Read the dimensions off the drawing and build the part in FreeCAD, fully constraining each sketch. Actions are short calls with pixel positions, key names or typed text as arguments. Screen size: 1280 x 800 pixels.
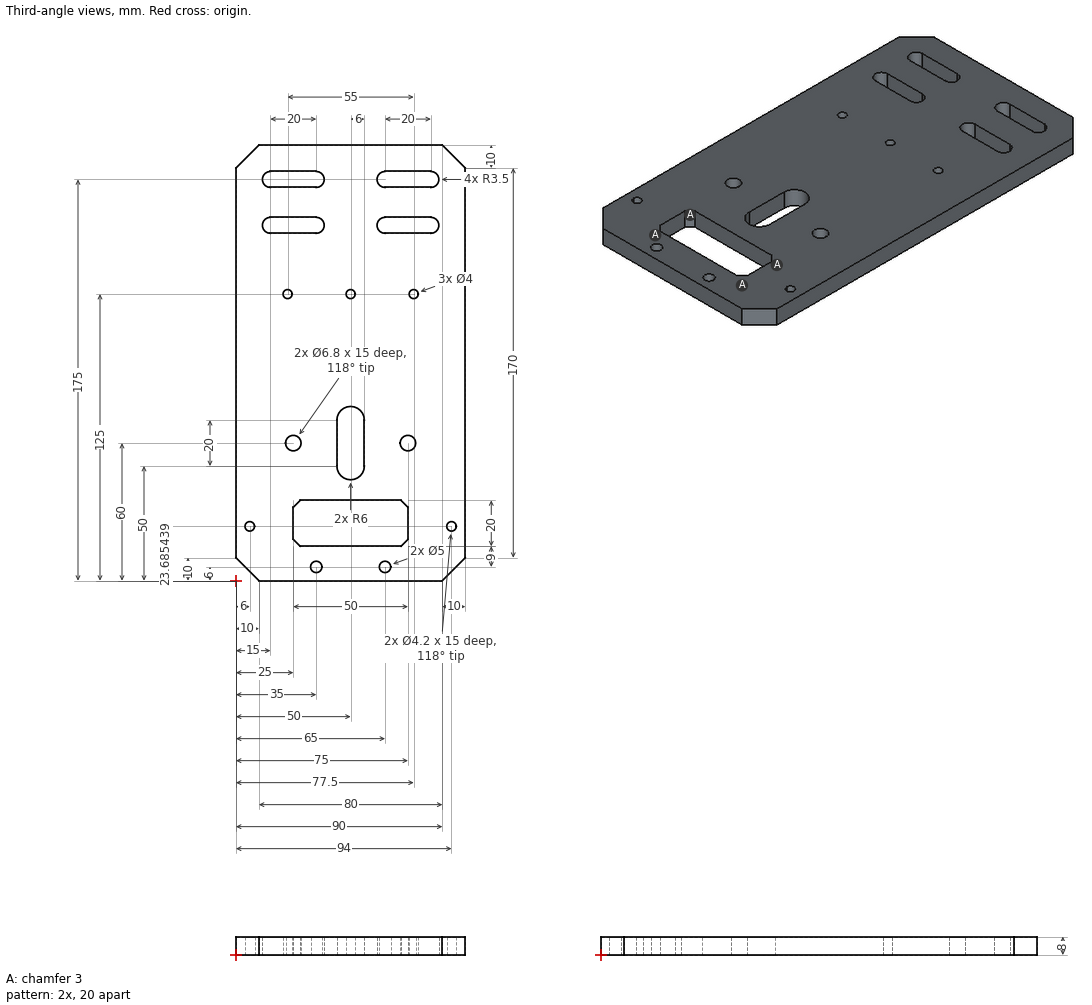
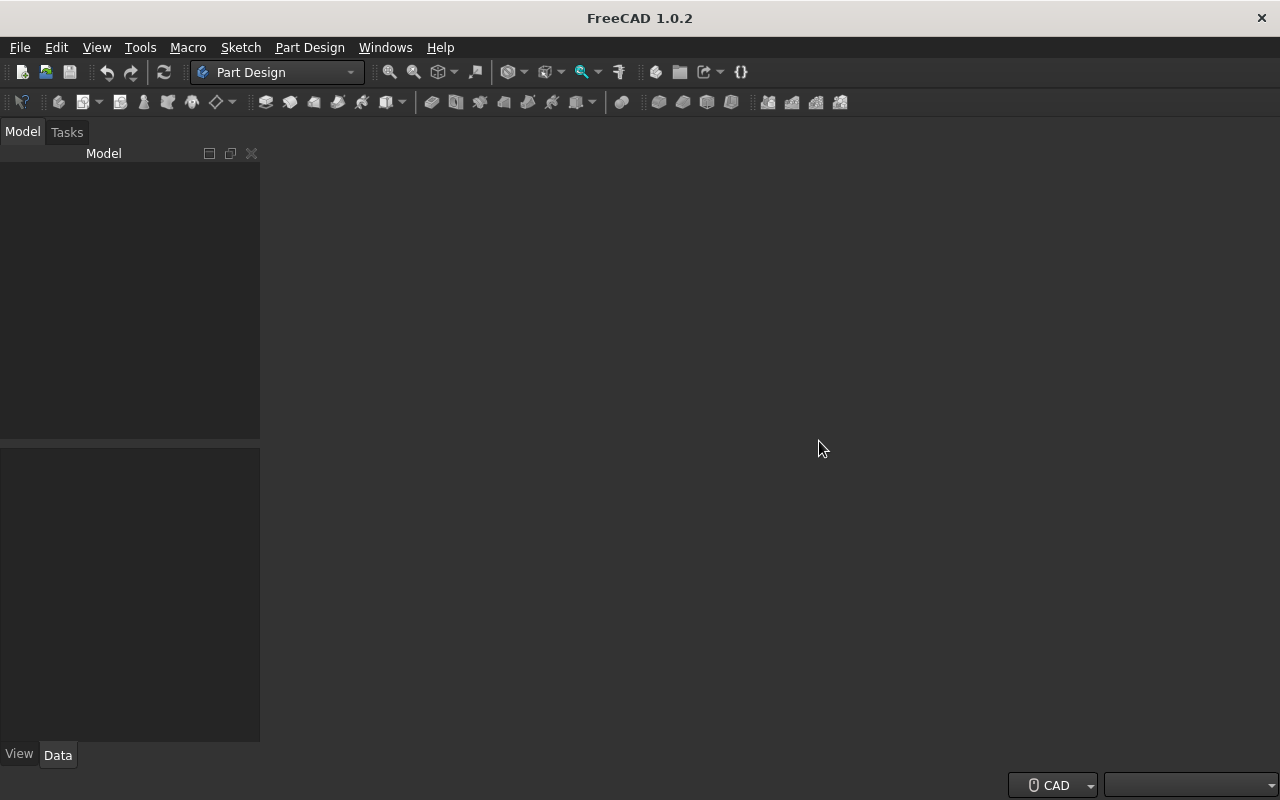
click(22, 72)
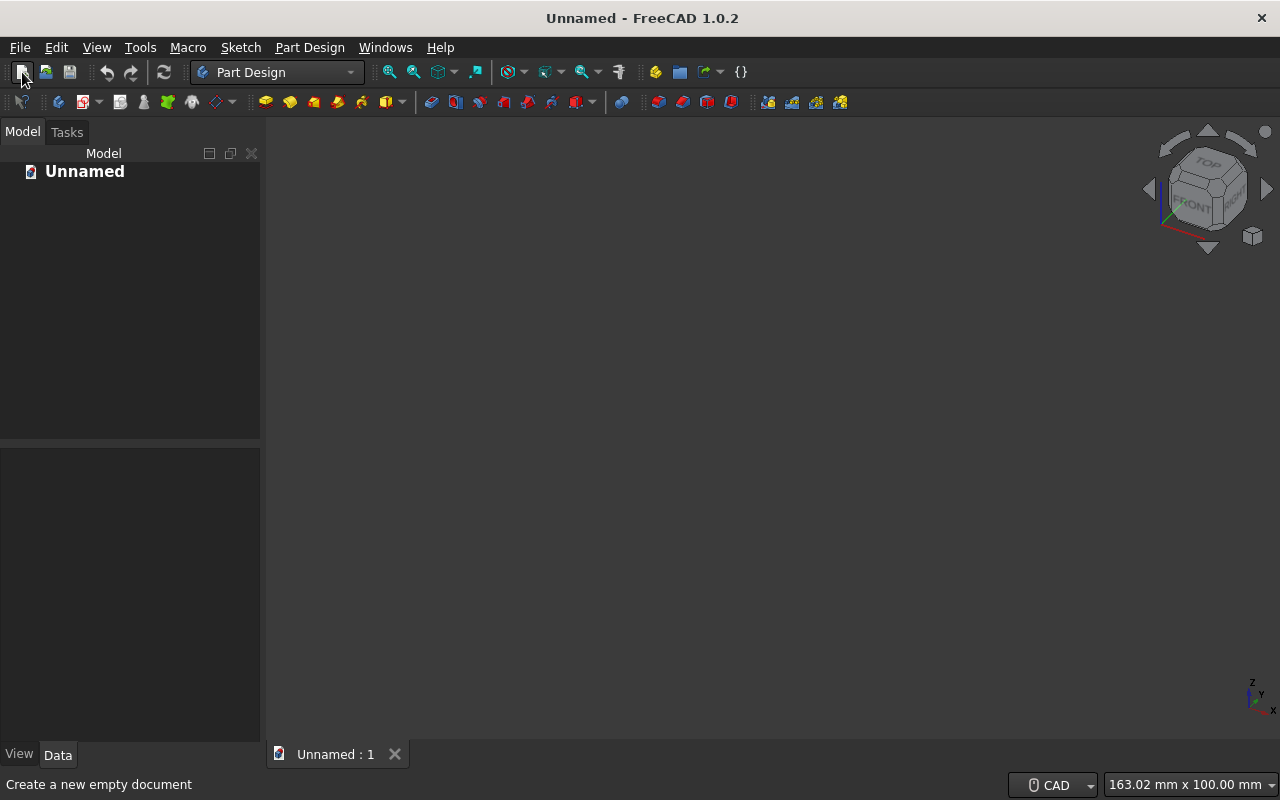
click(84, 102)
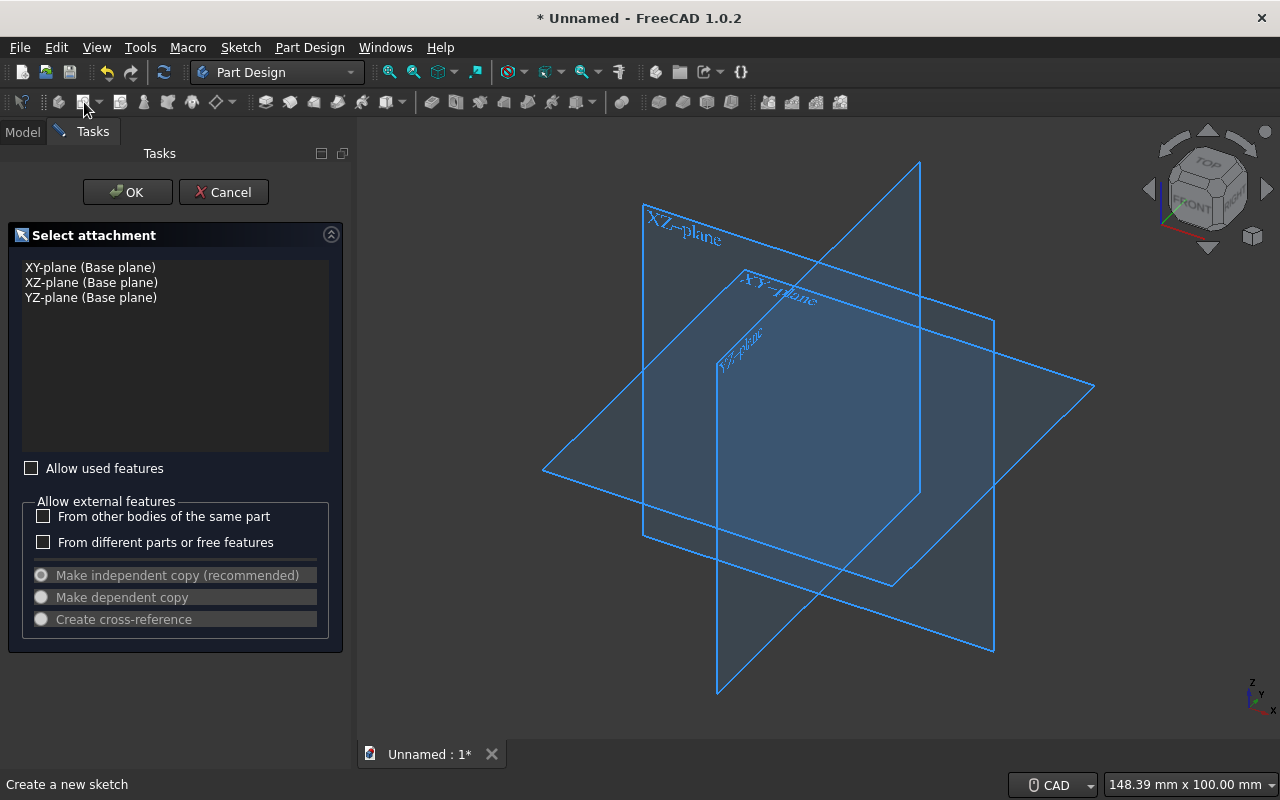
click(82, 268)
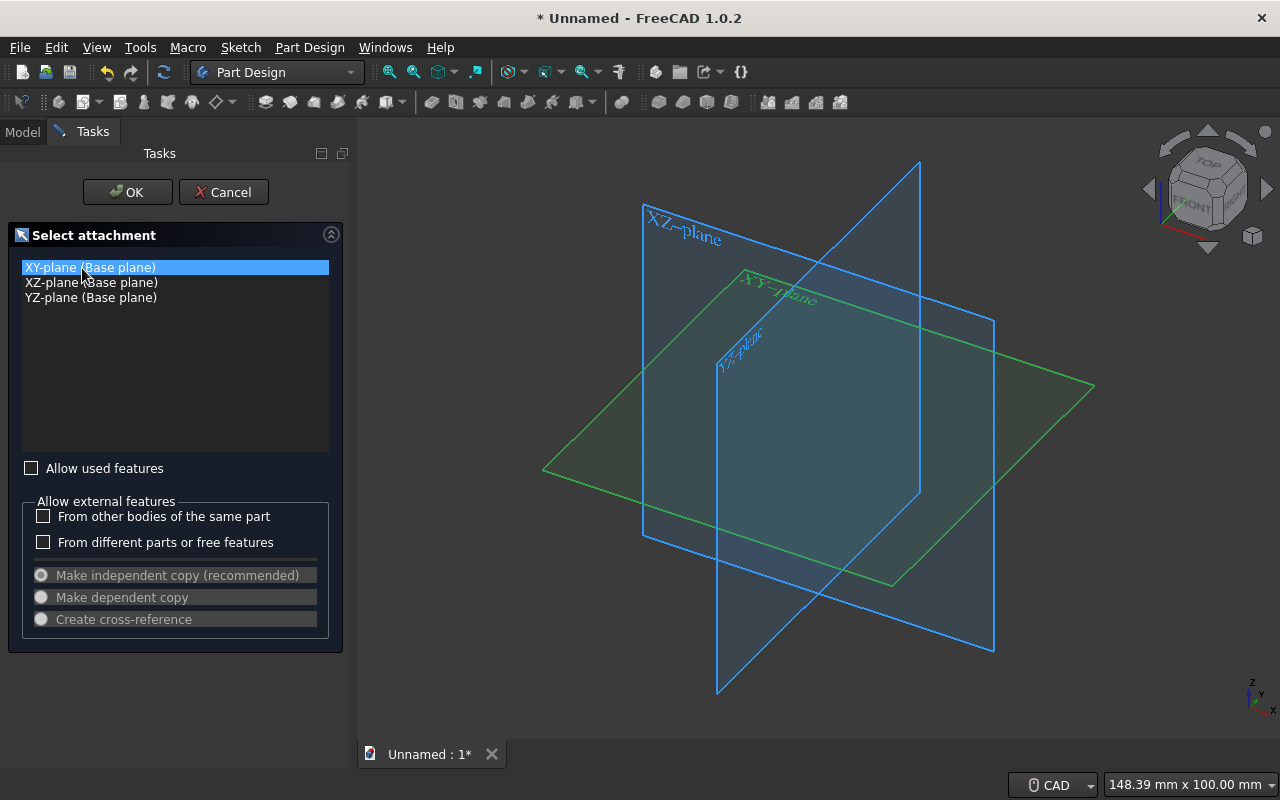
click(128, 192)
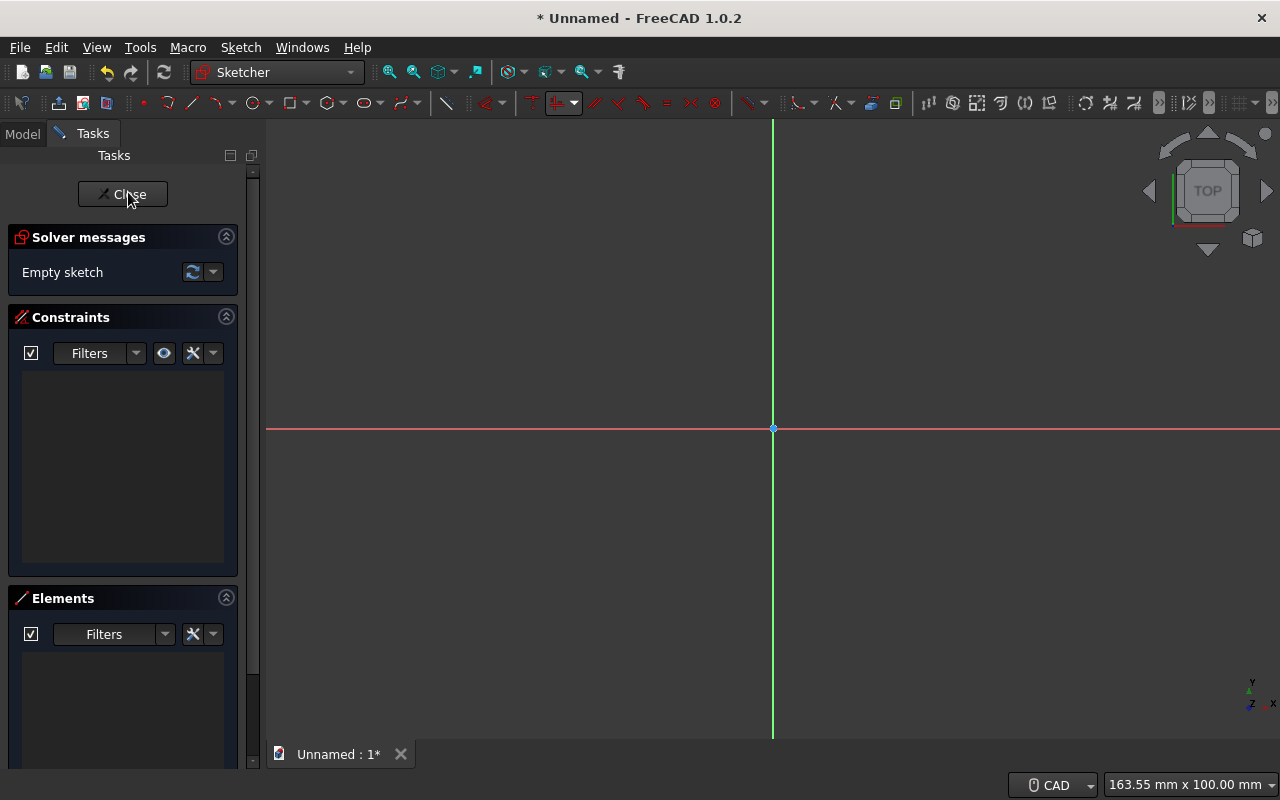
scroll(484, 711, down, 5)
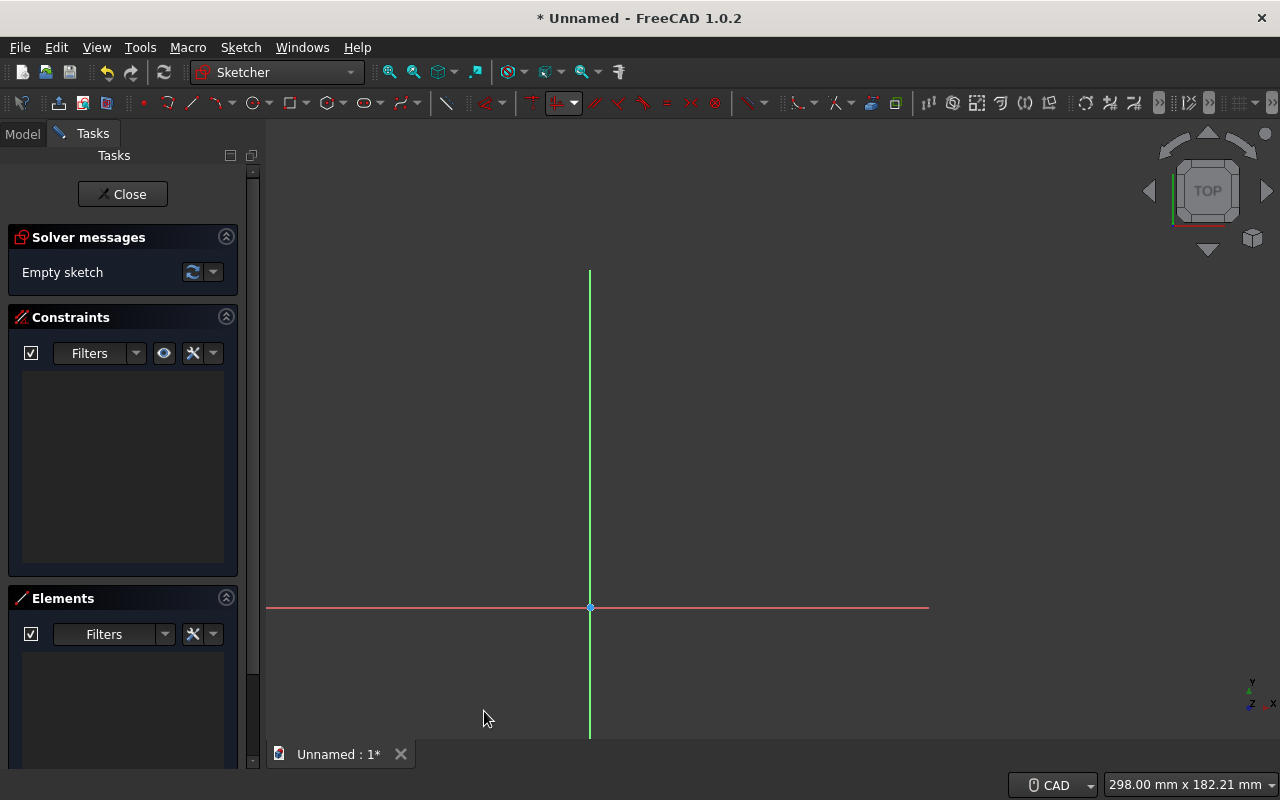
key(g)
key(m)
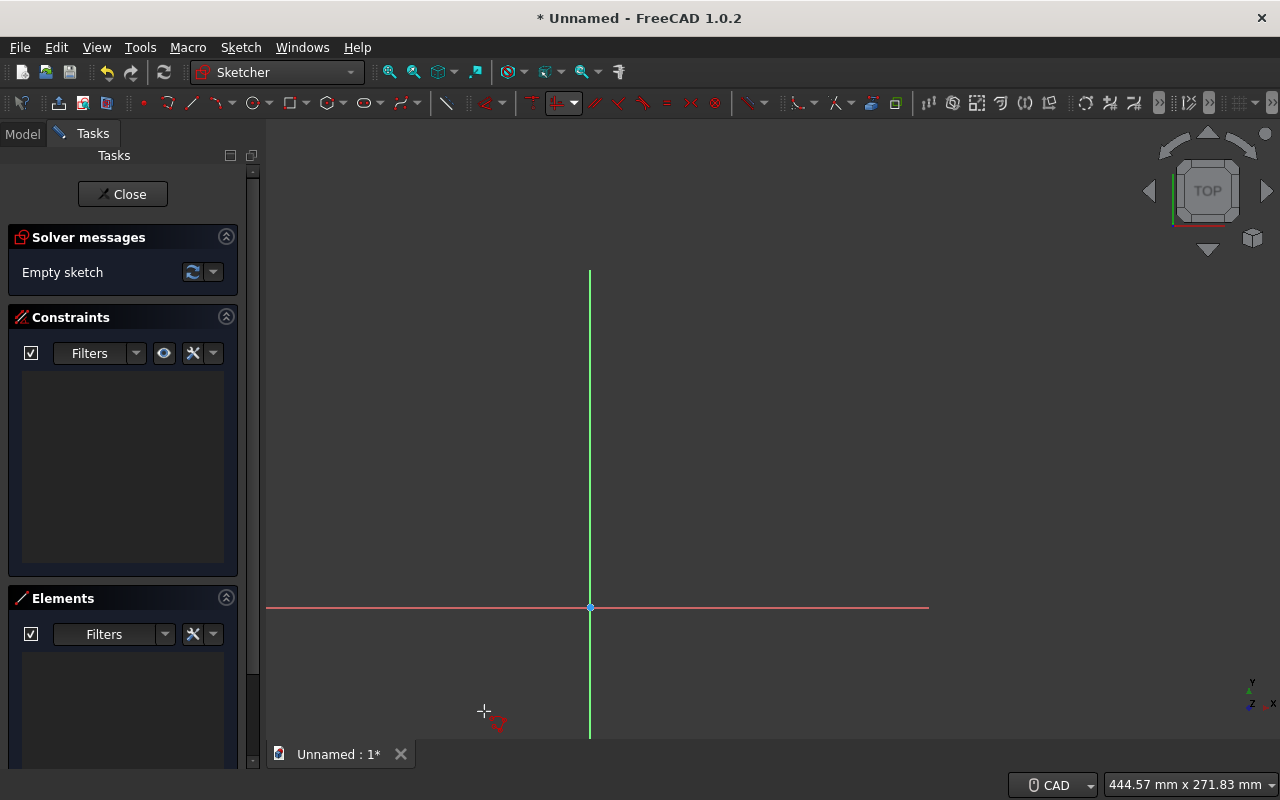
click(590, 585)
click(613, 608)
click(796, 599)
click(819, 585)
click(819, 197)
click(796, 175)
click(613, 175)
click(599, 197)
click(590, 586)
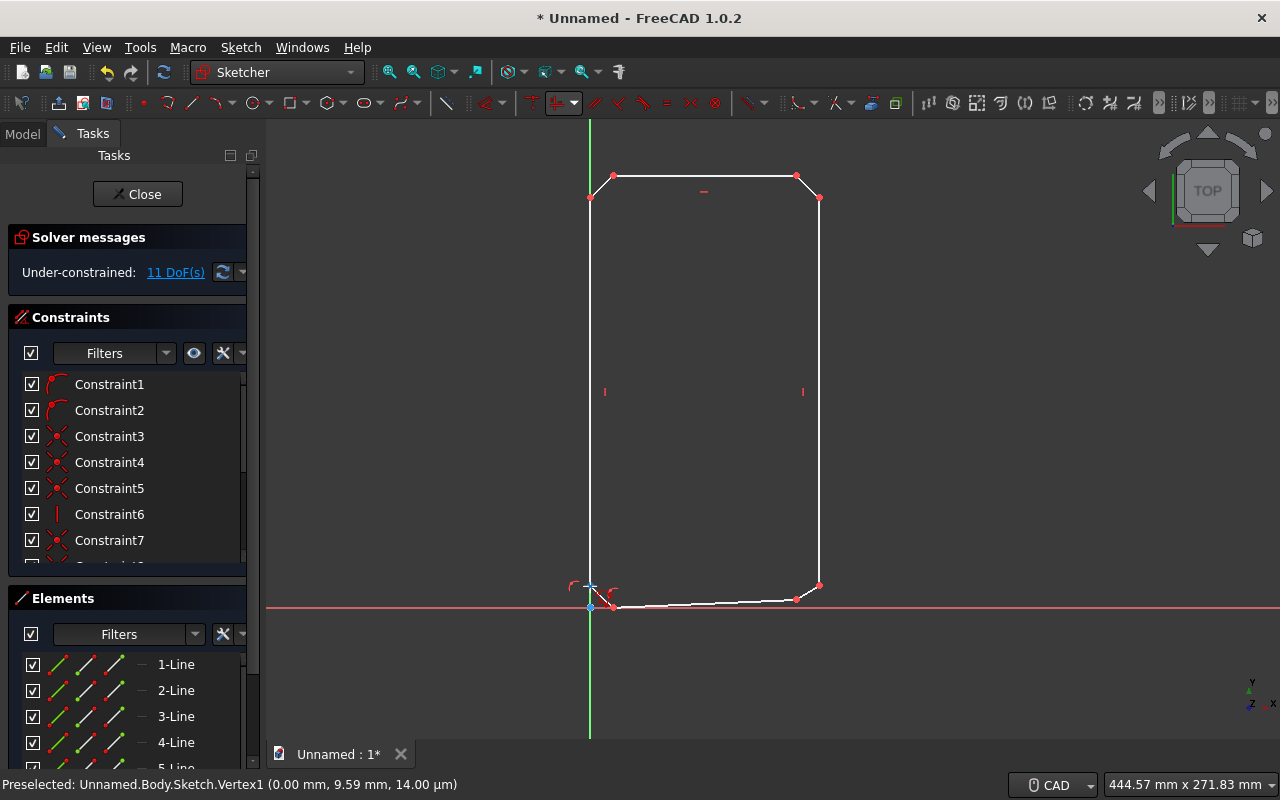
click(290, 104)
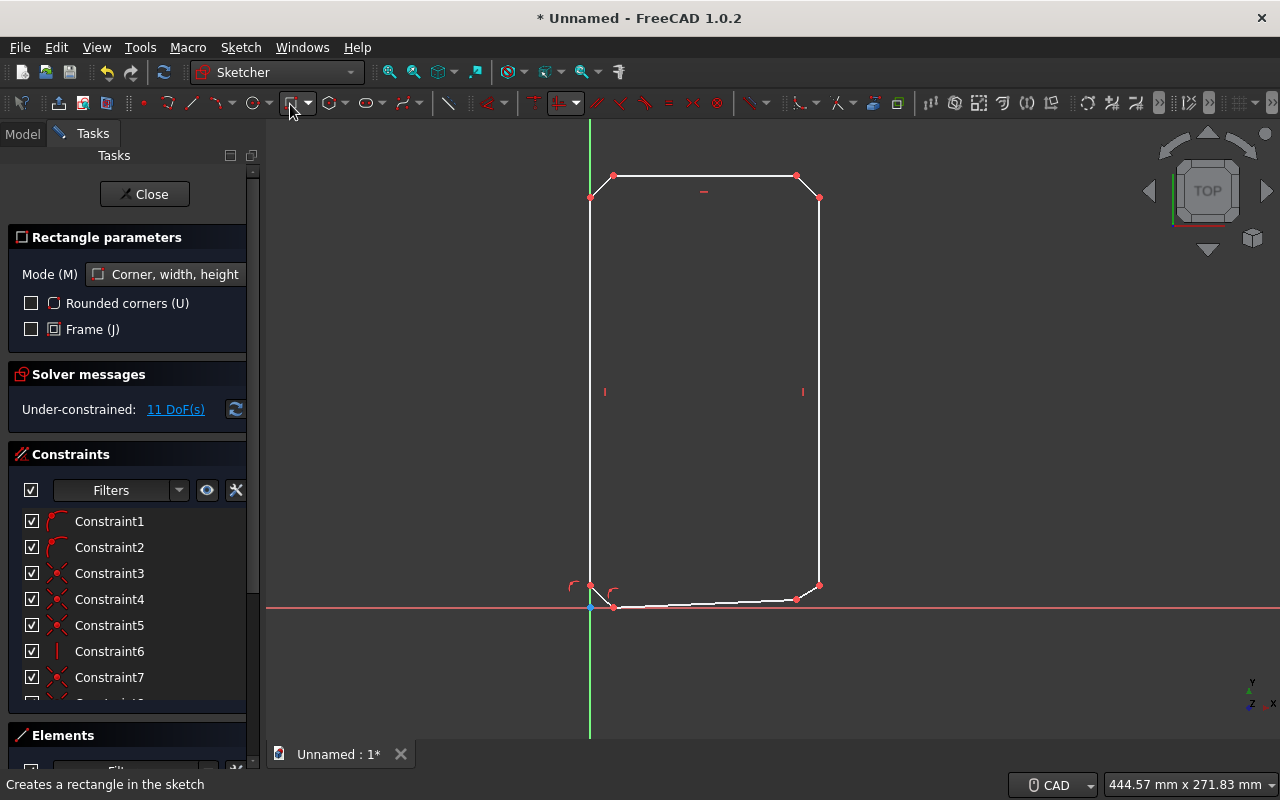
click(647, 528)
move(762, 574)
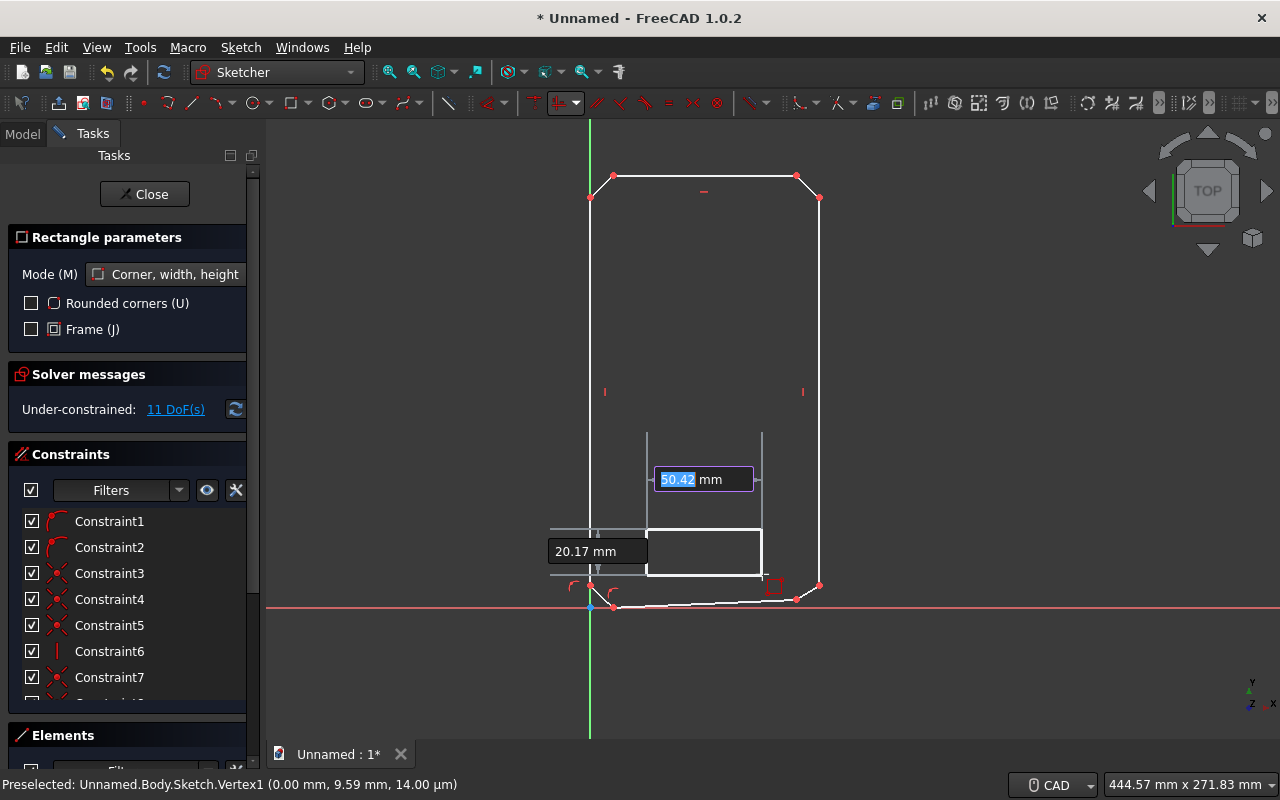
text(50)
key(Tab)
text(20)
key(Return)